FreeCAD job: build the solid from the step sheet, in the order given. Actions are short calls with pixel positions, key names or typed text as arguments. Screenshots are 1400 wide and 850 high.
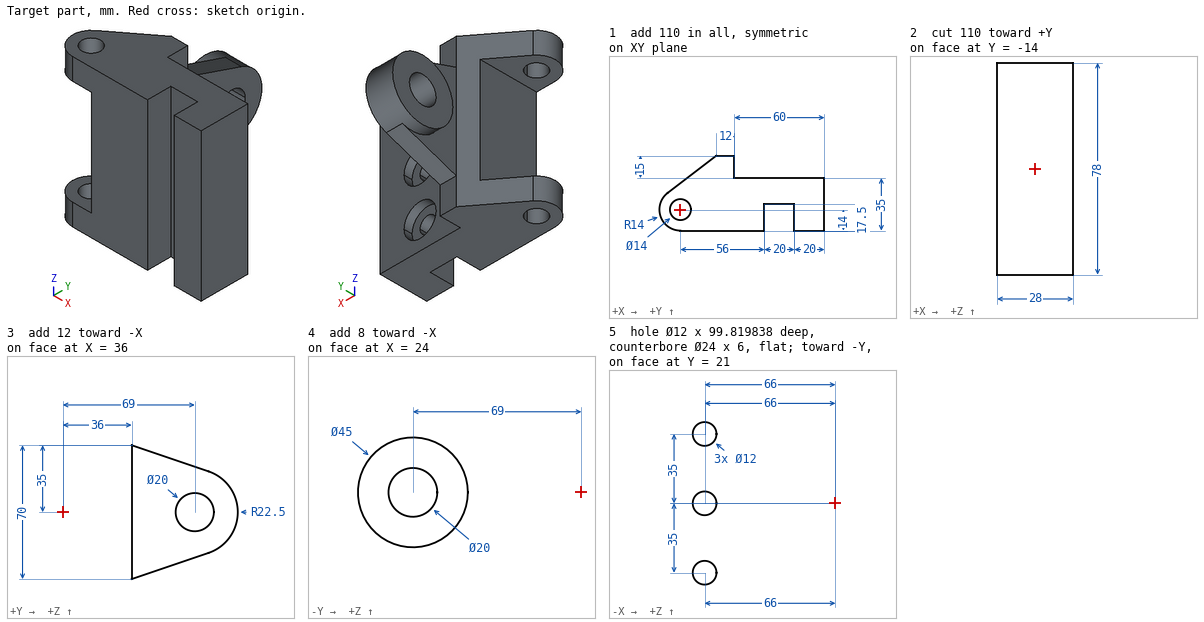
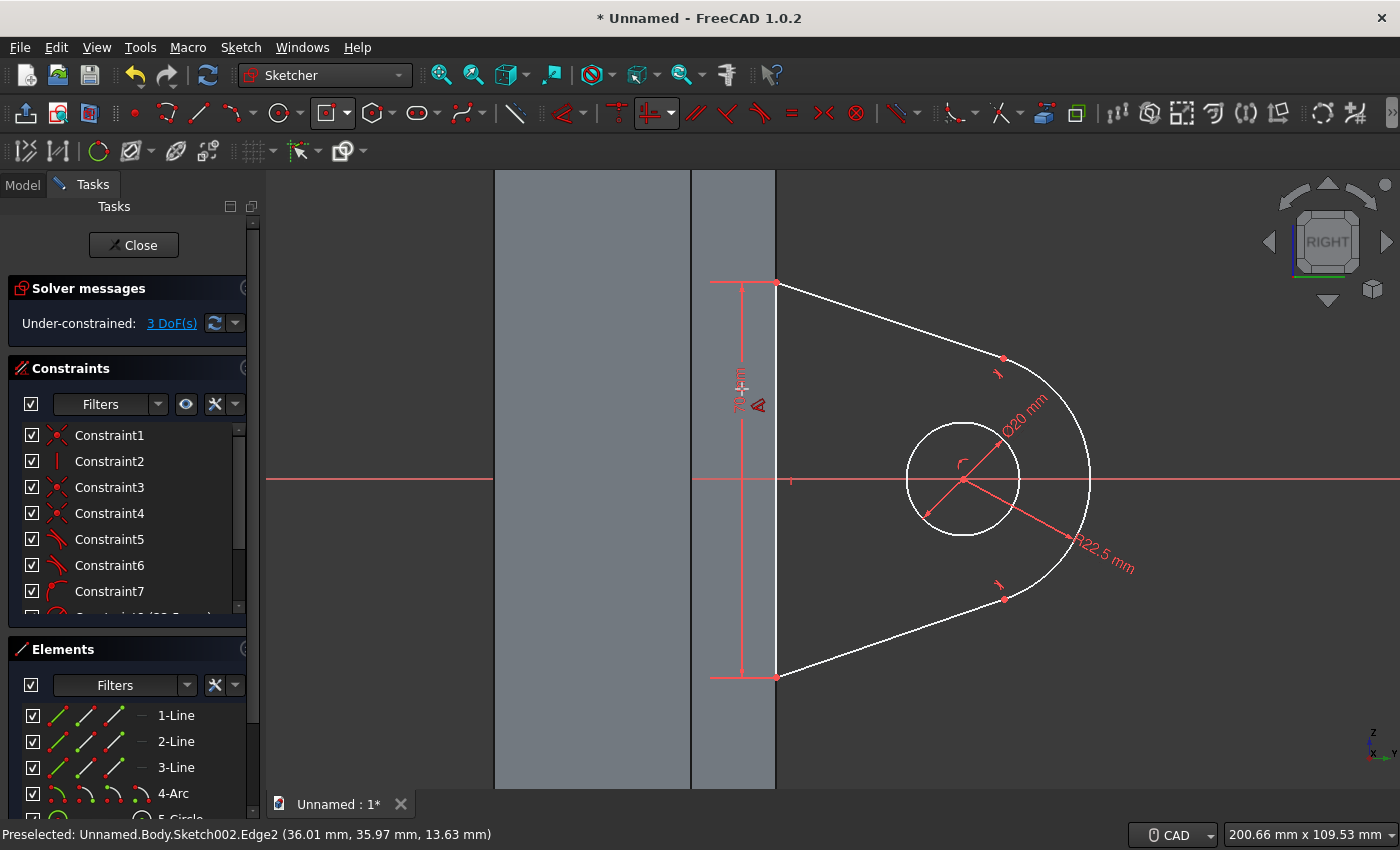
click(963, 479)
click(678, 513)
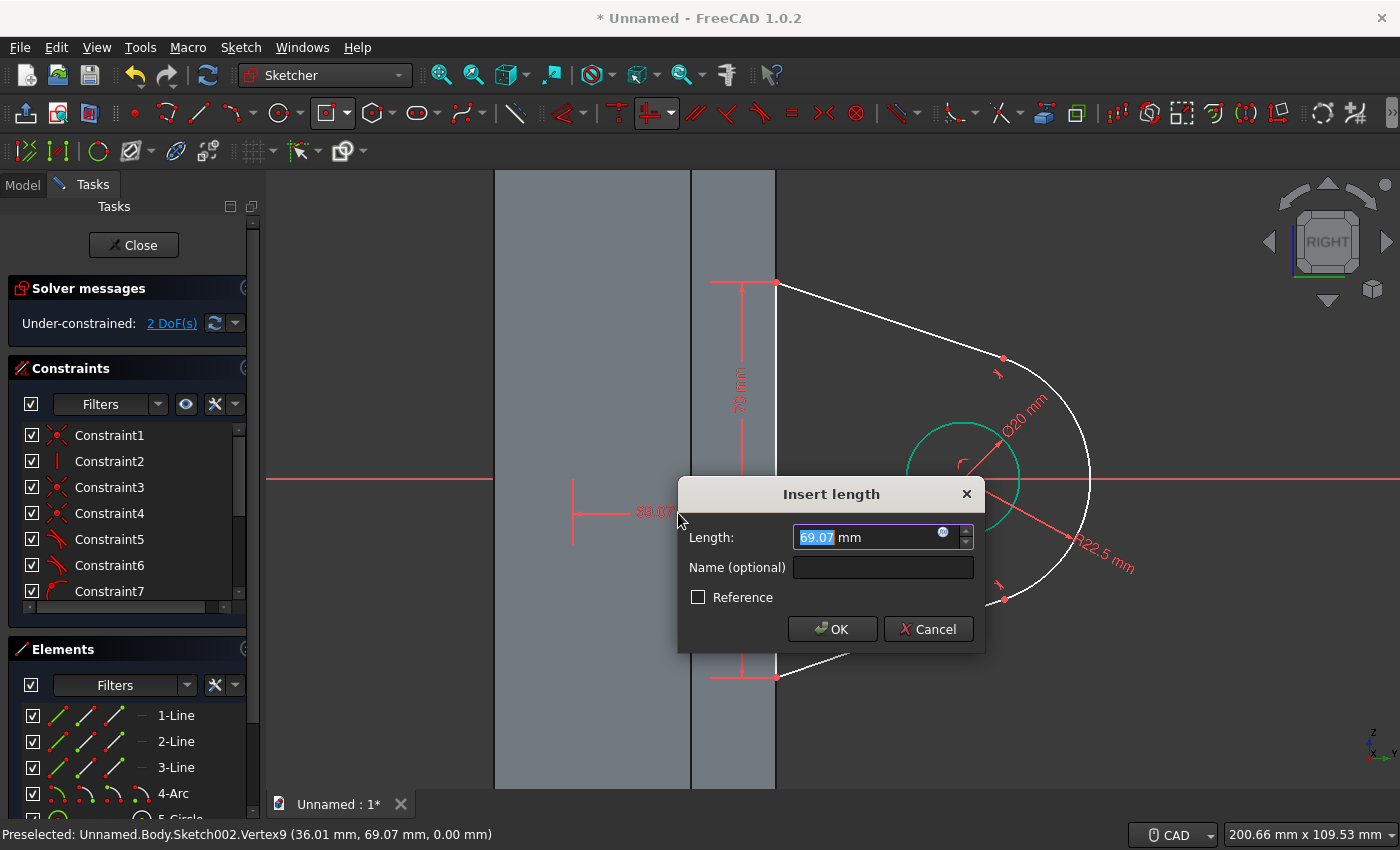
text(69)
key(Return)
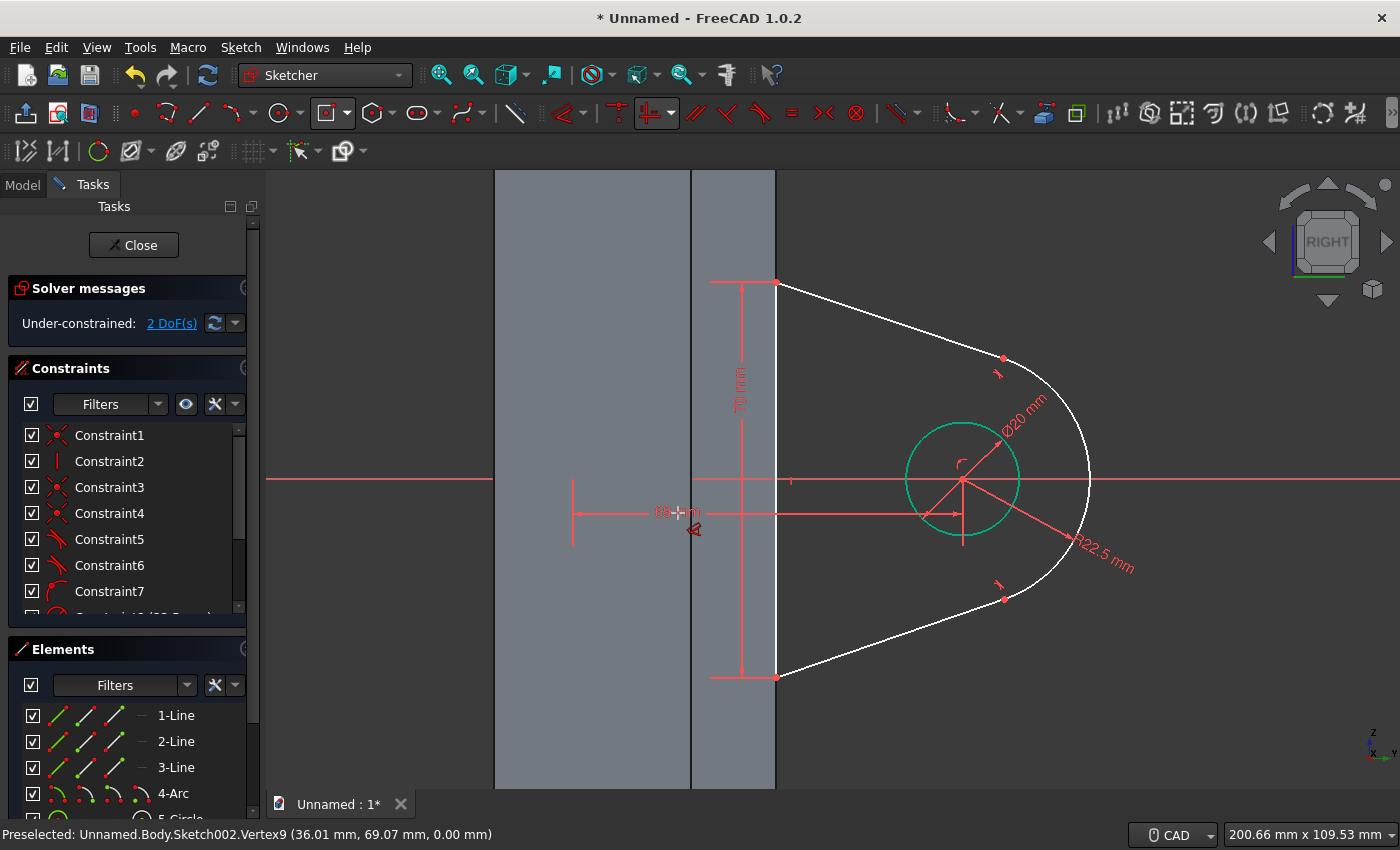
click(776, 282)
click(674, 248)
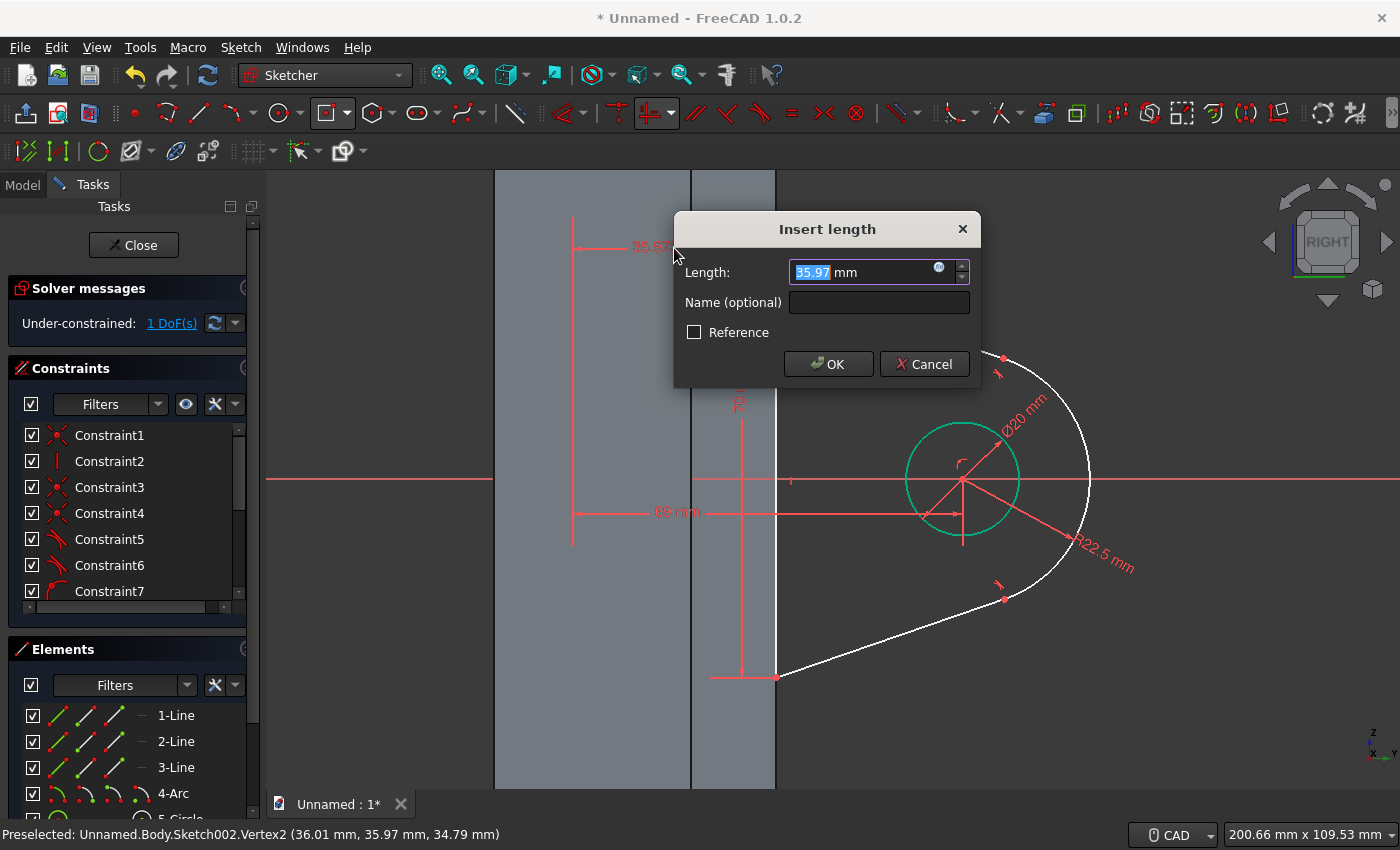
text(36)
key(Return)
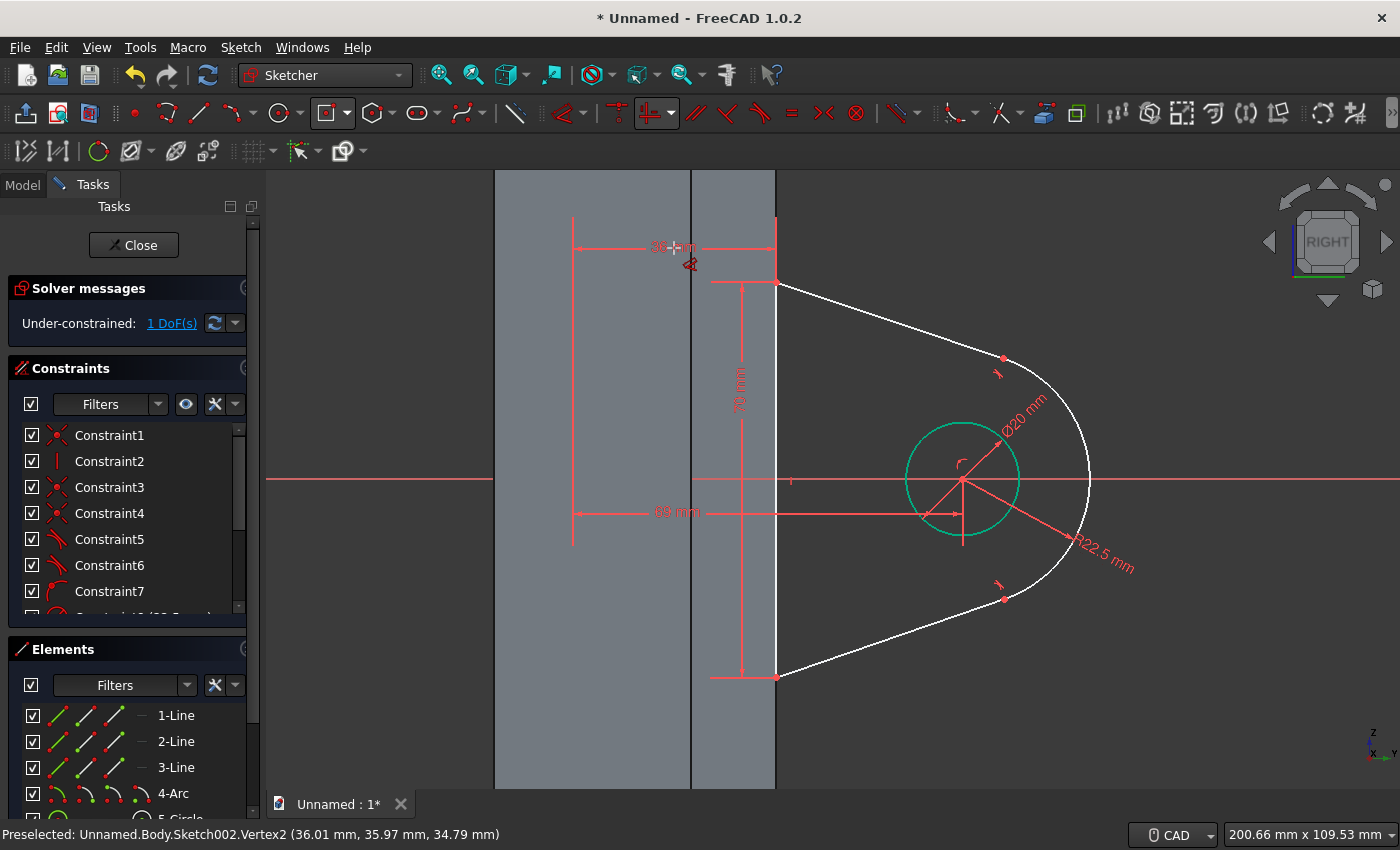
click(776, 282)
click(539, 381)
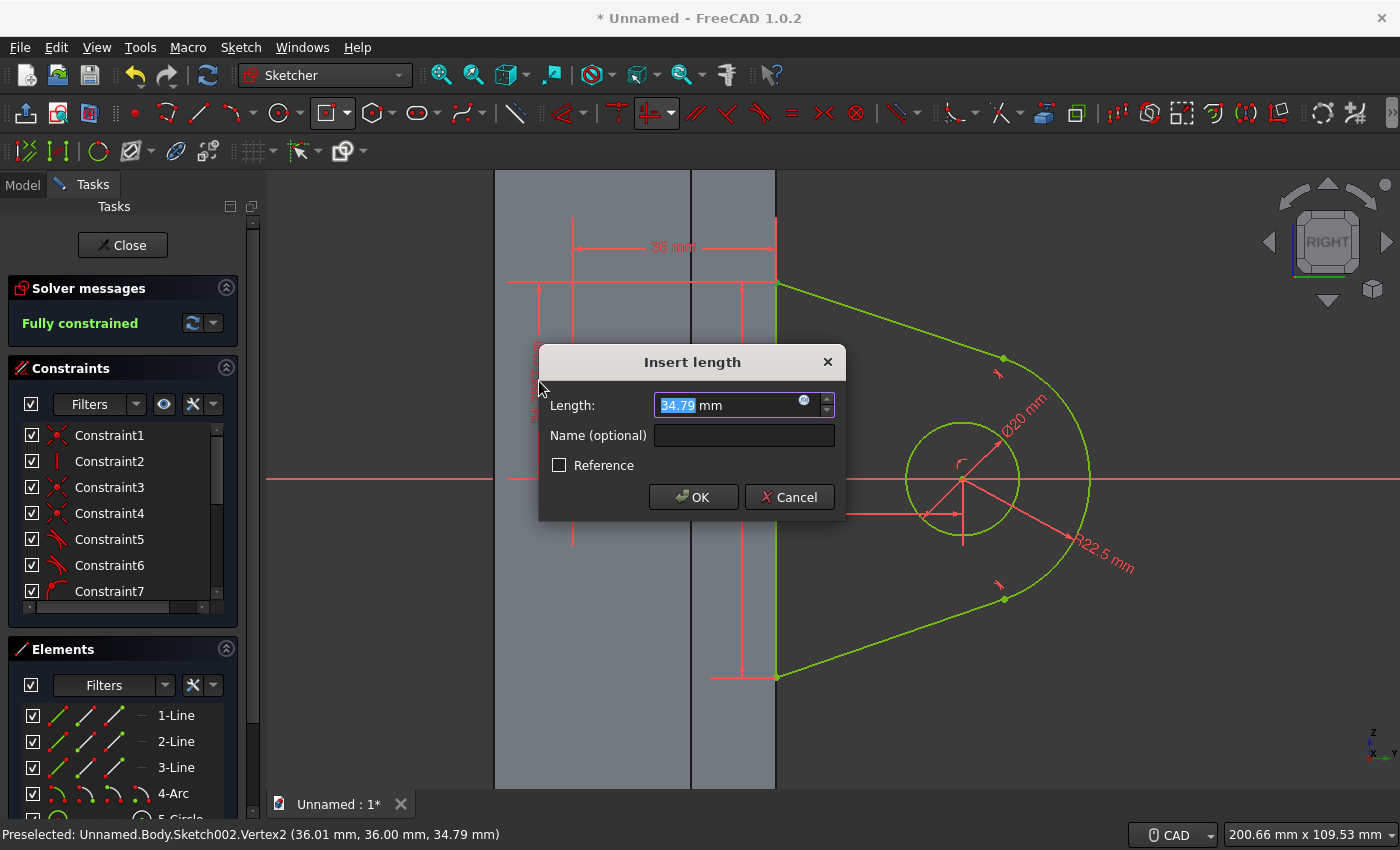
text(35)
key(Return)
key(Escape)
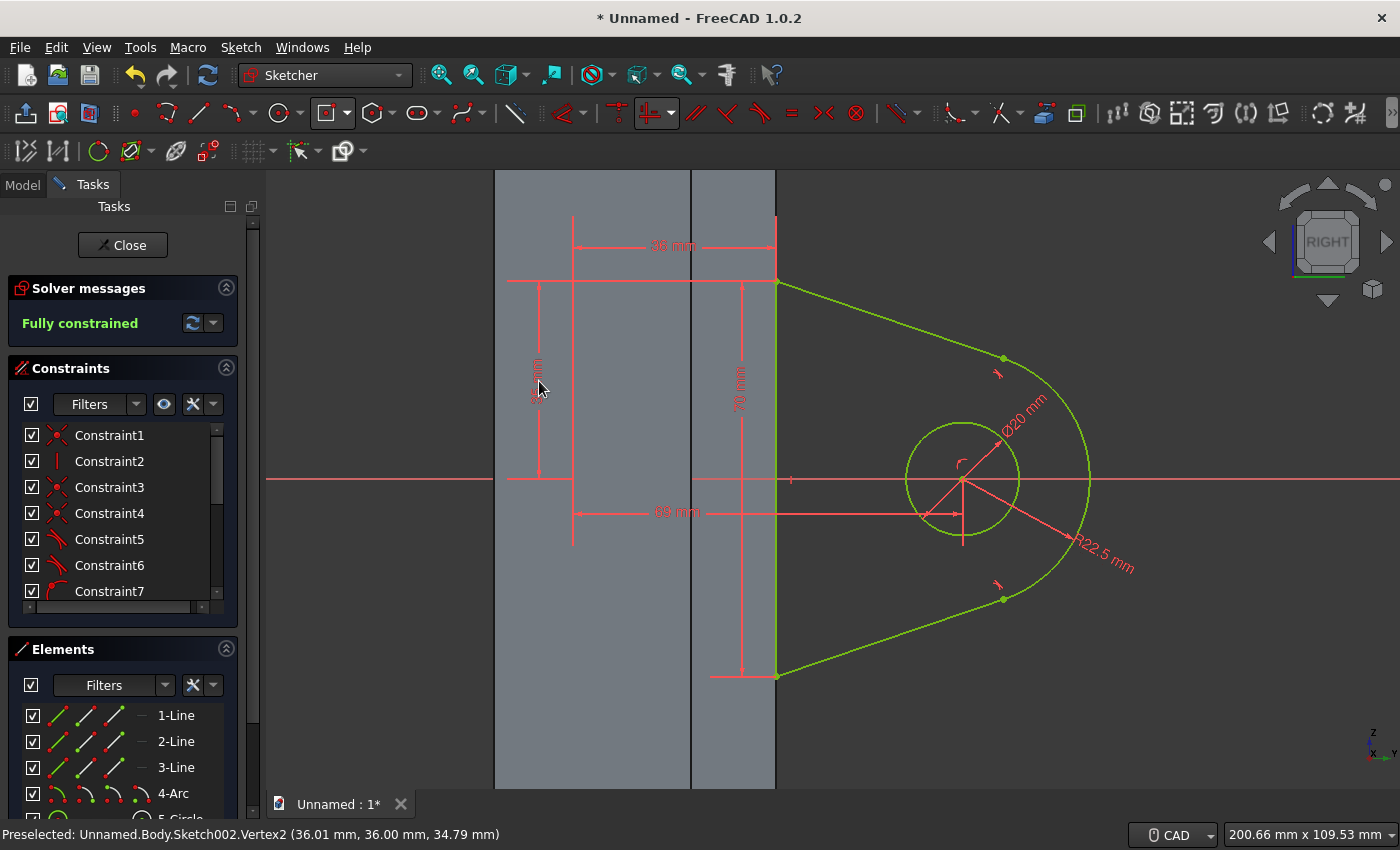
click(123, 245)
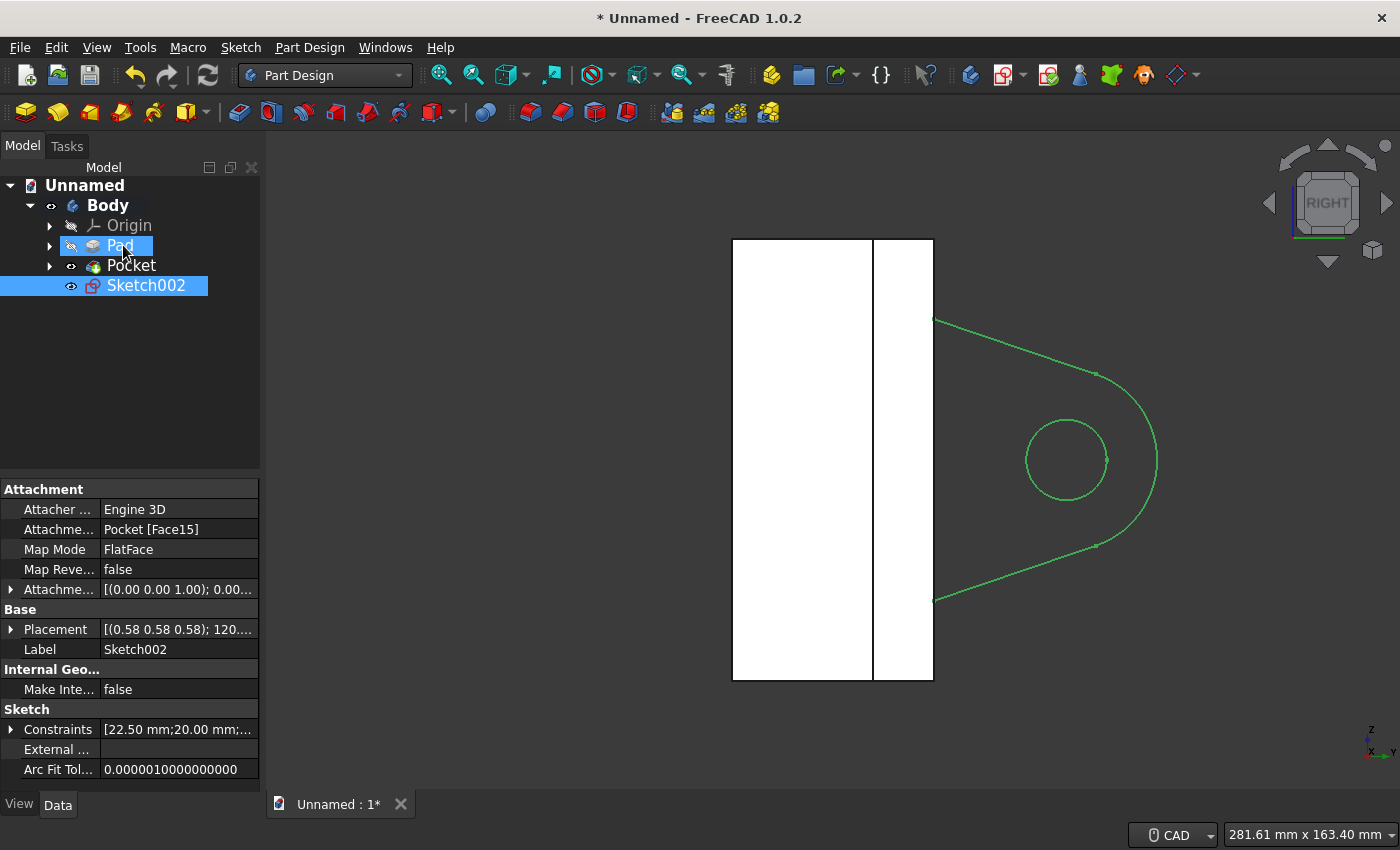
click(26, 112)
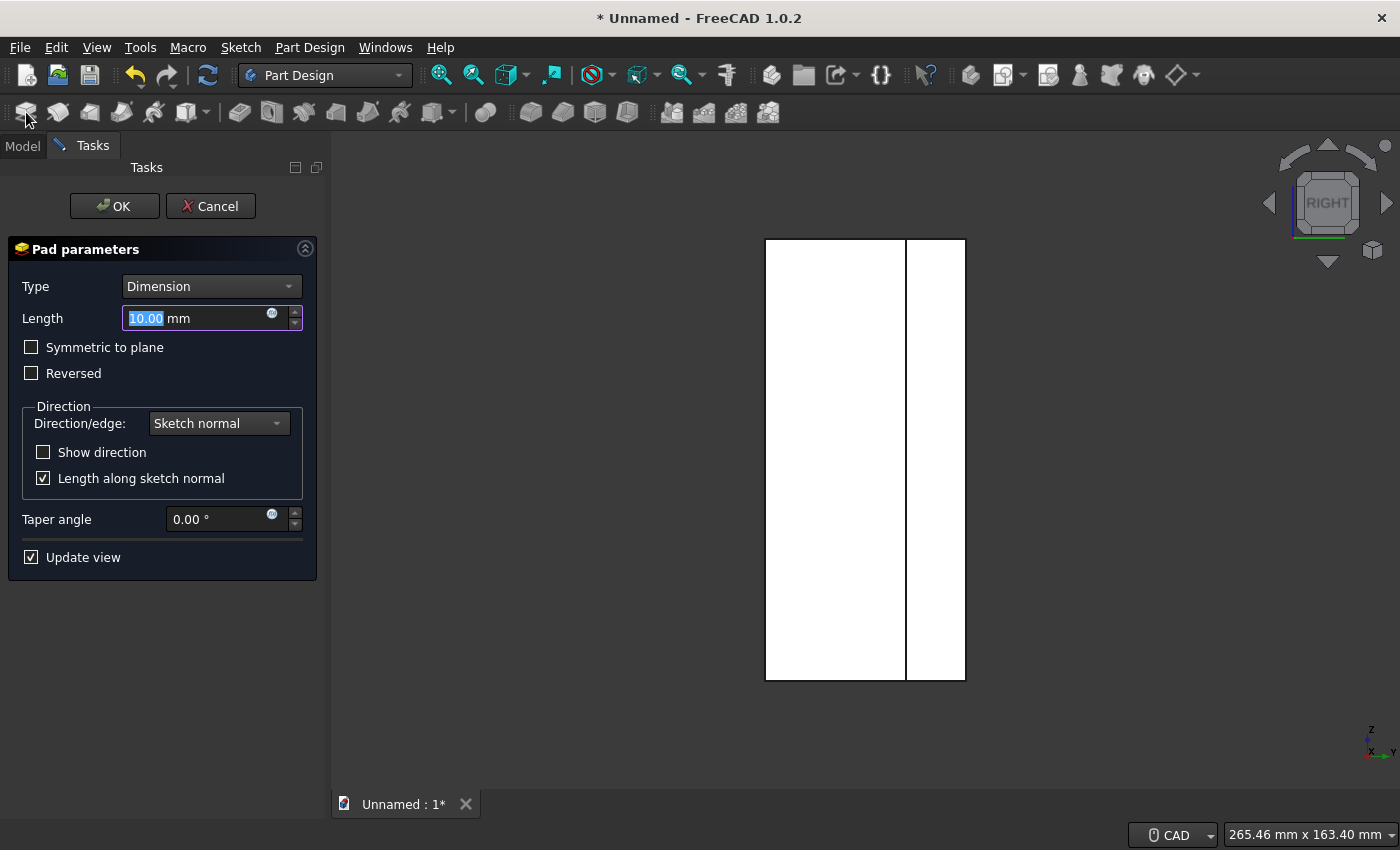
text(12)
key(Tab)